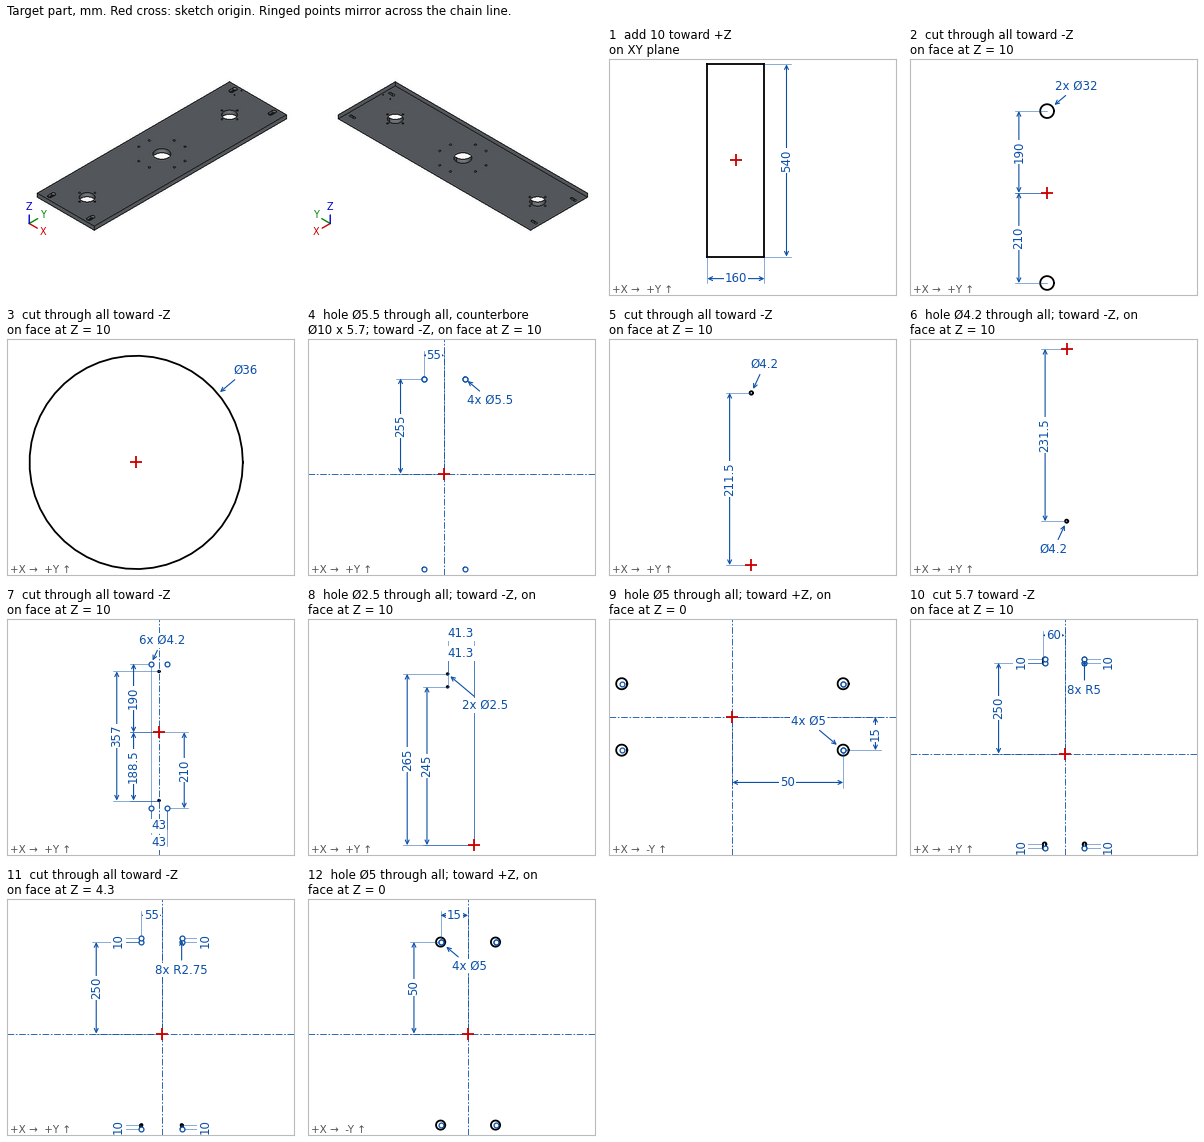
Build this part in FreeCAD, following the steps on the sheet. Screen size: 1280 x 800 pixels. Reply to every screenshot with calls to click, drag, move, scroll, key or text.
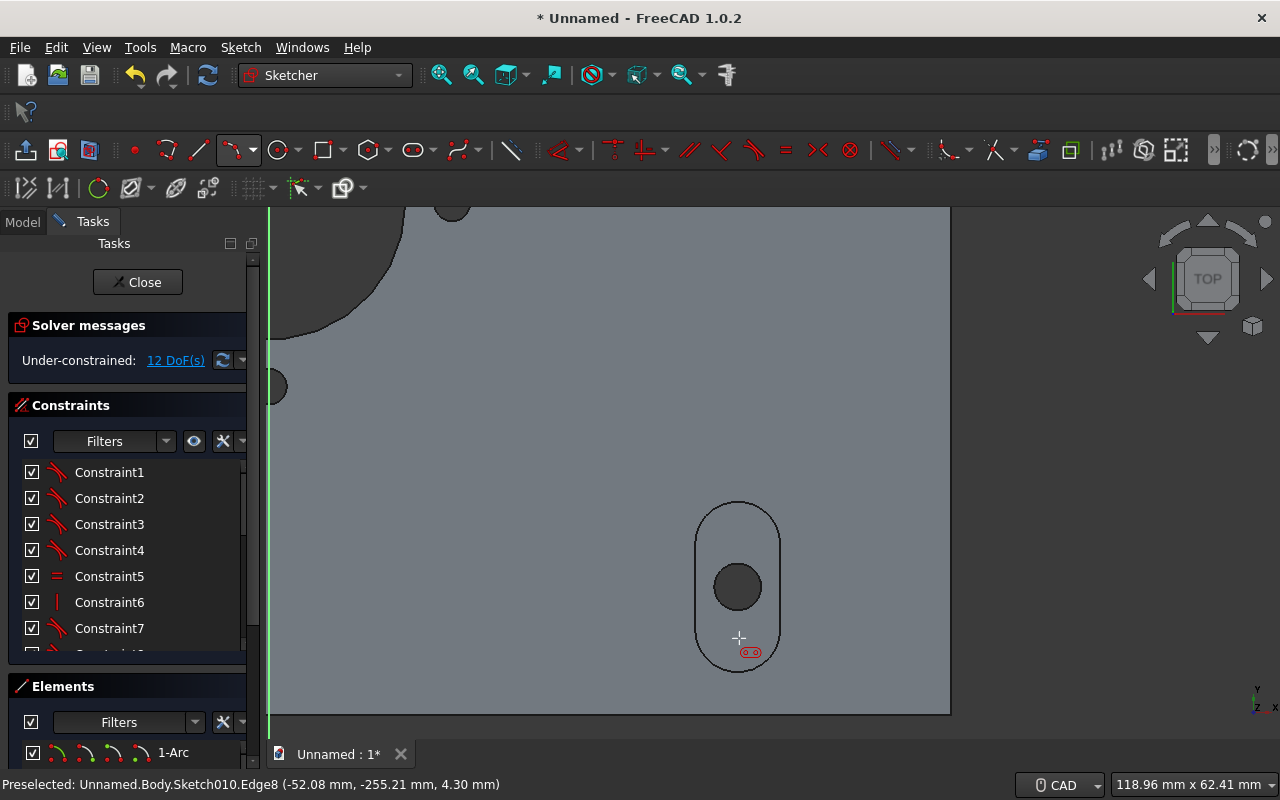
scroll(739, 638, down, 13)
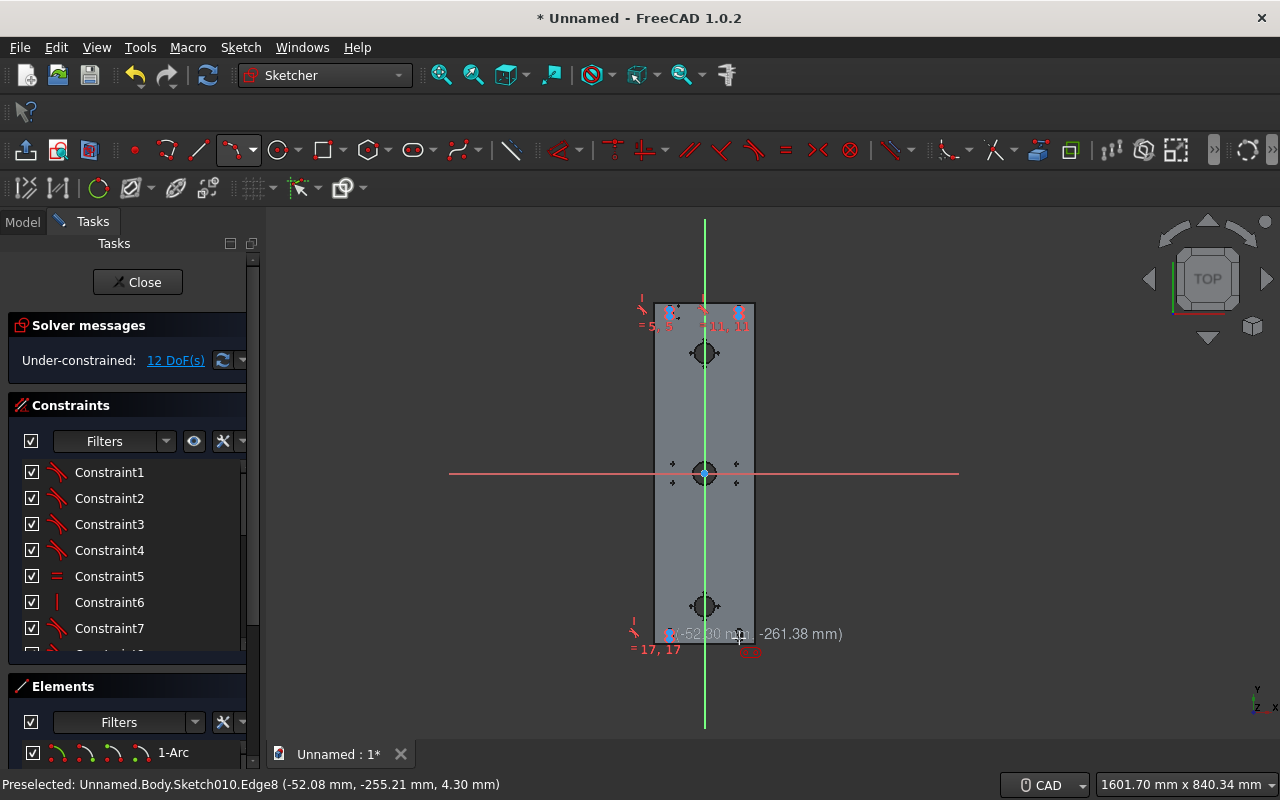
click(739, 638)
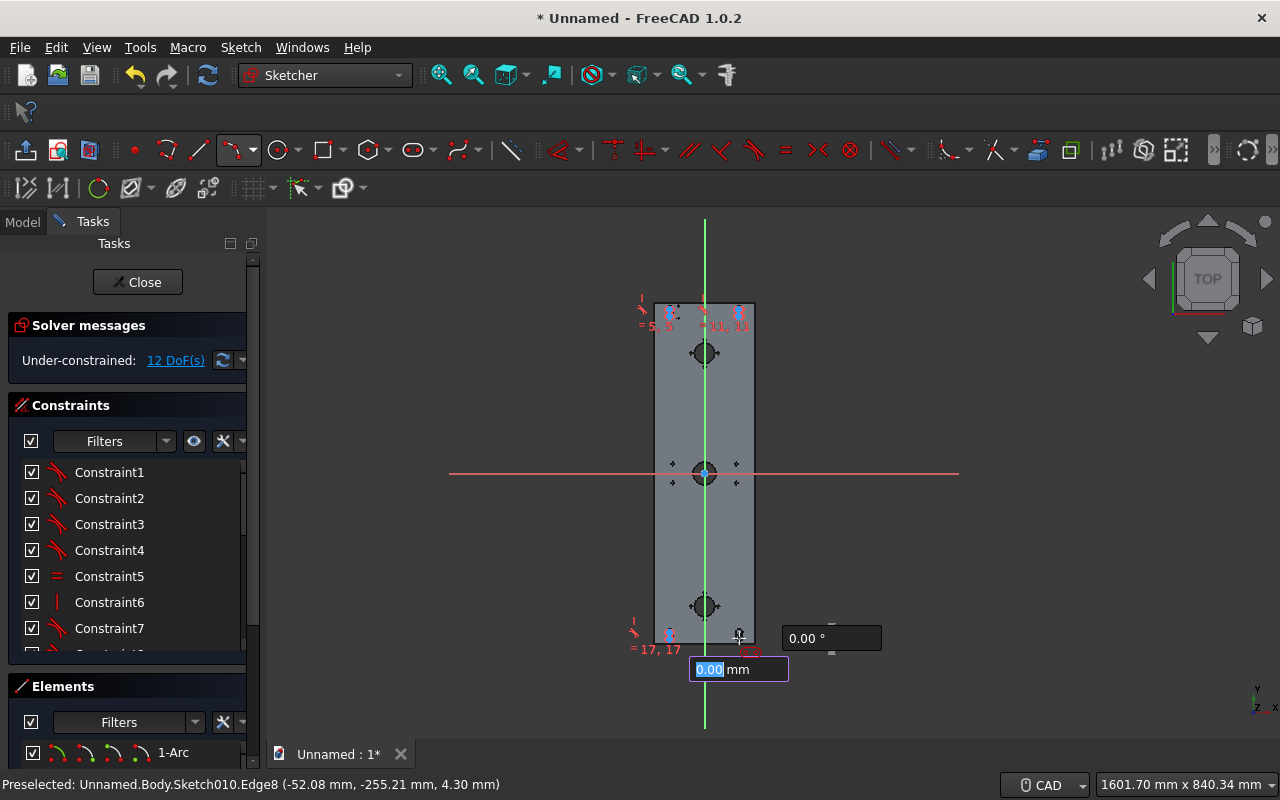
scroll(739, 632, up, 5)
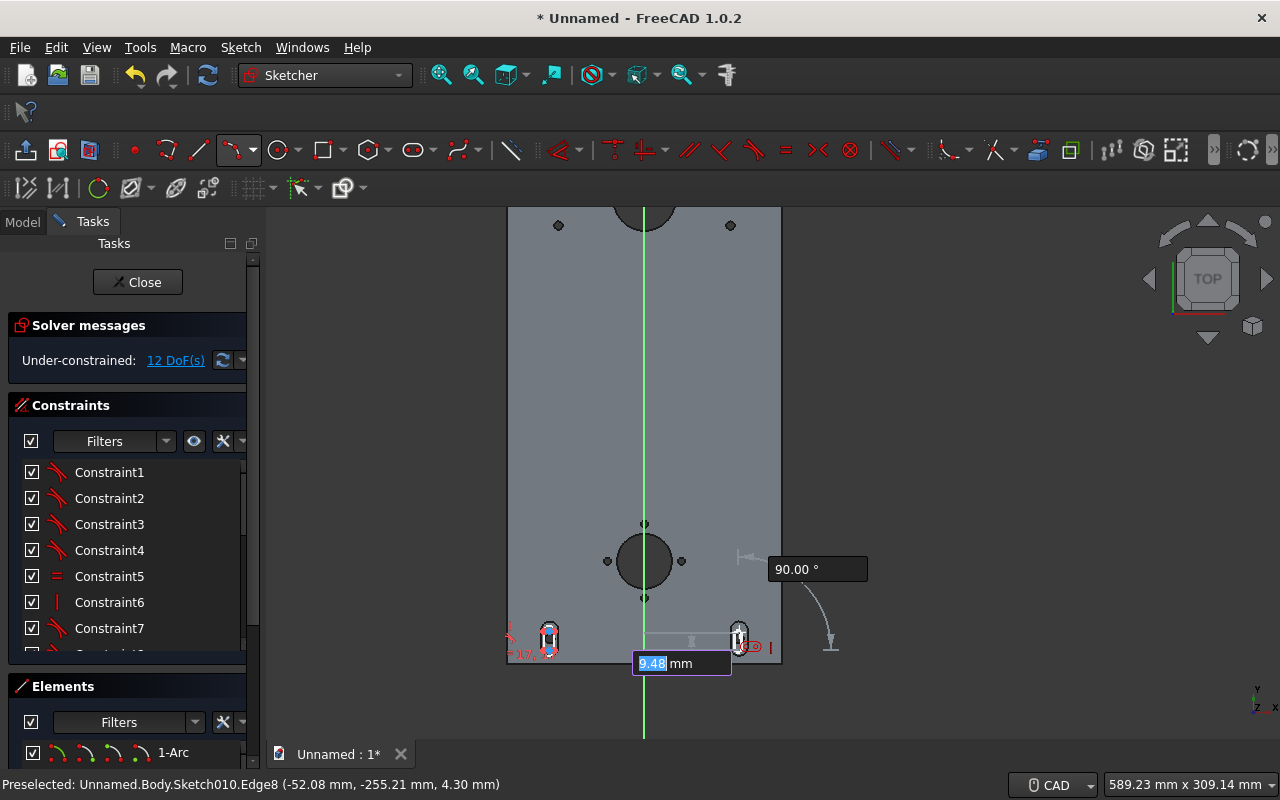
click(738, 630)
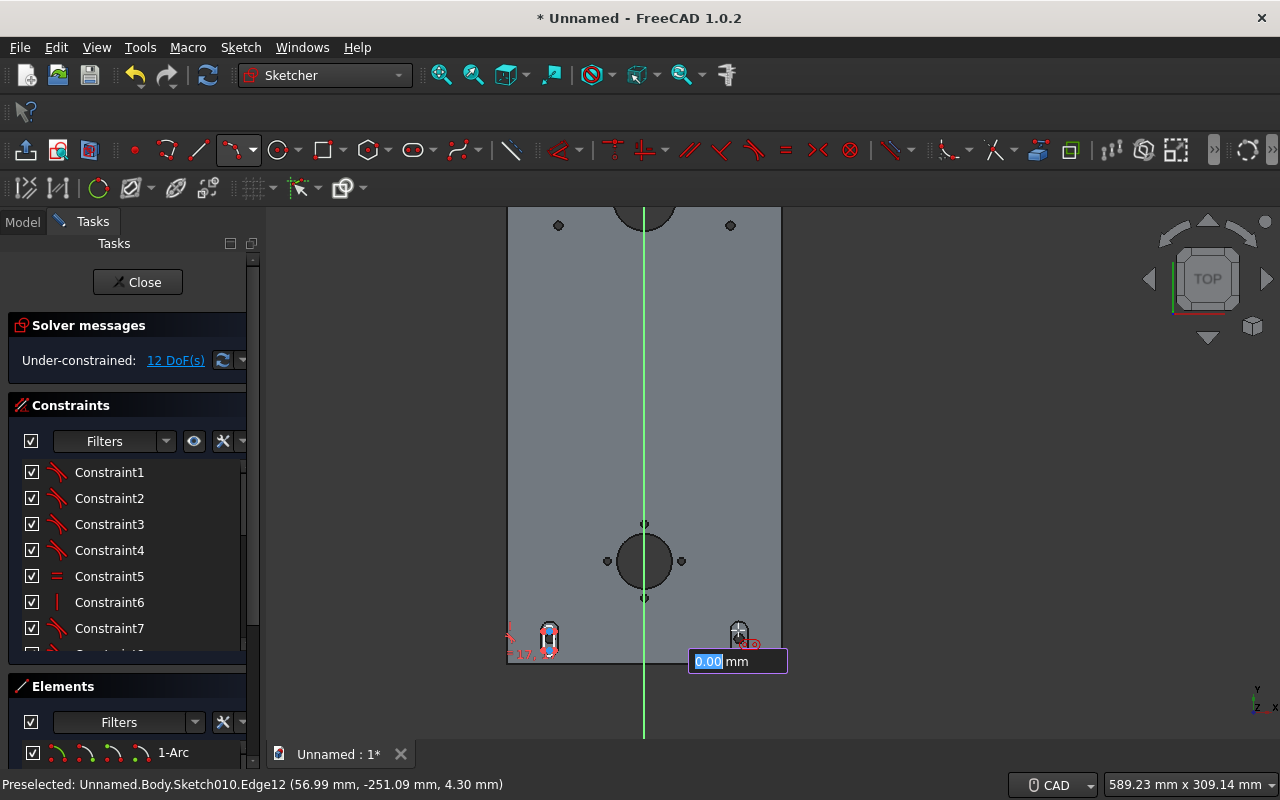
scroll(744, 639, up, 7)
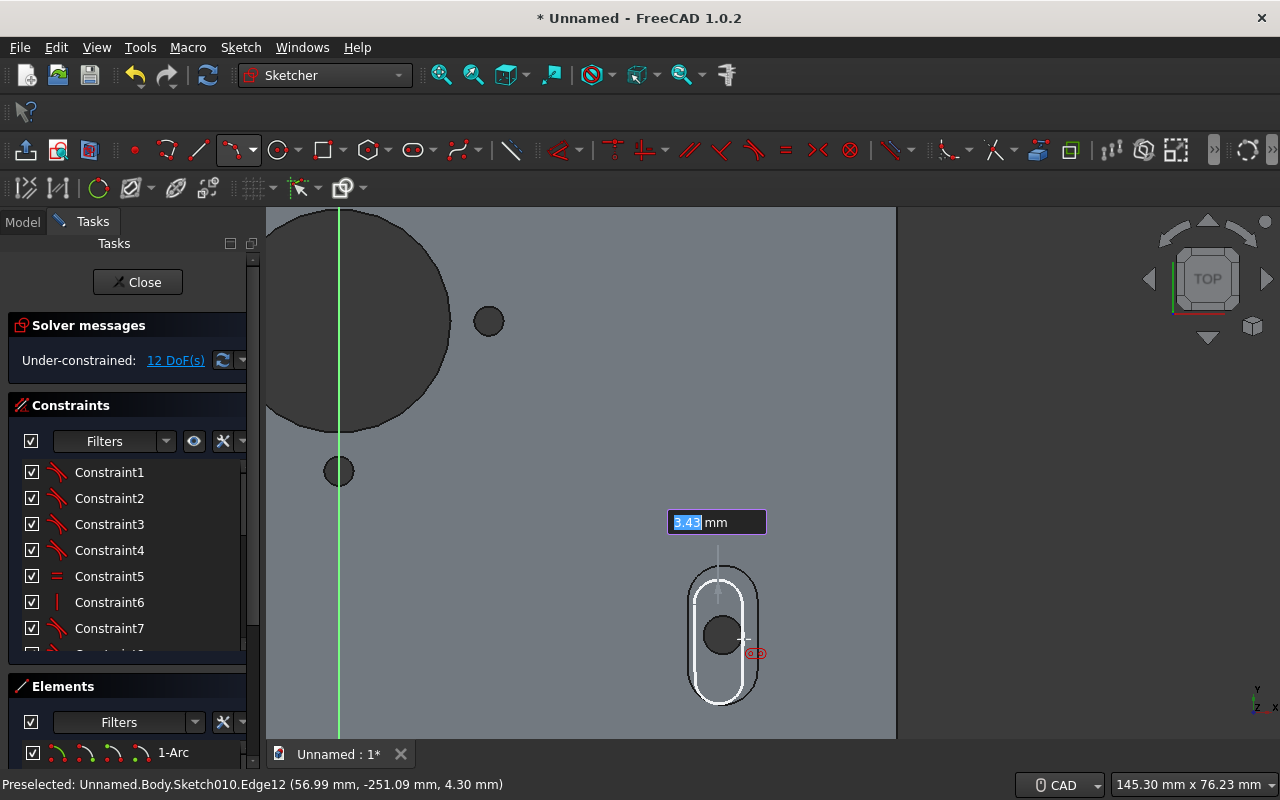
click(742, 635)
key(Escape)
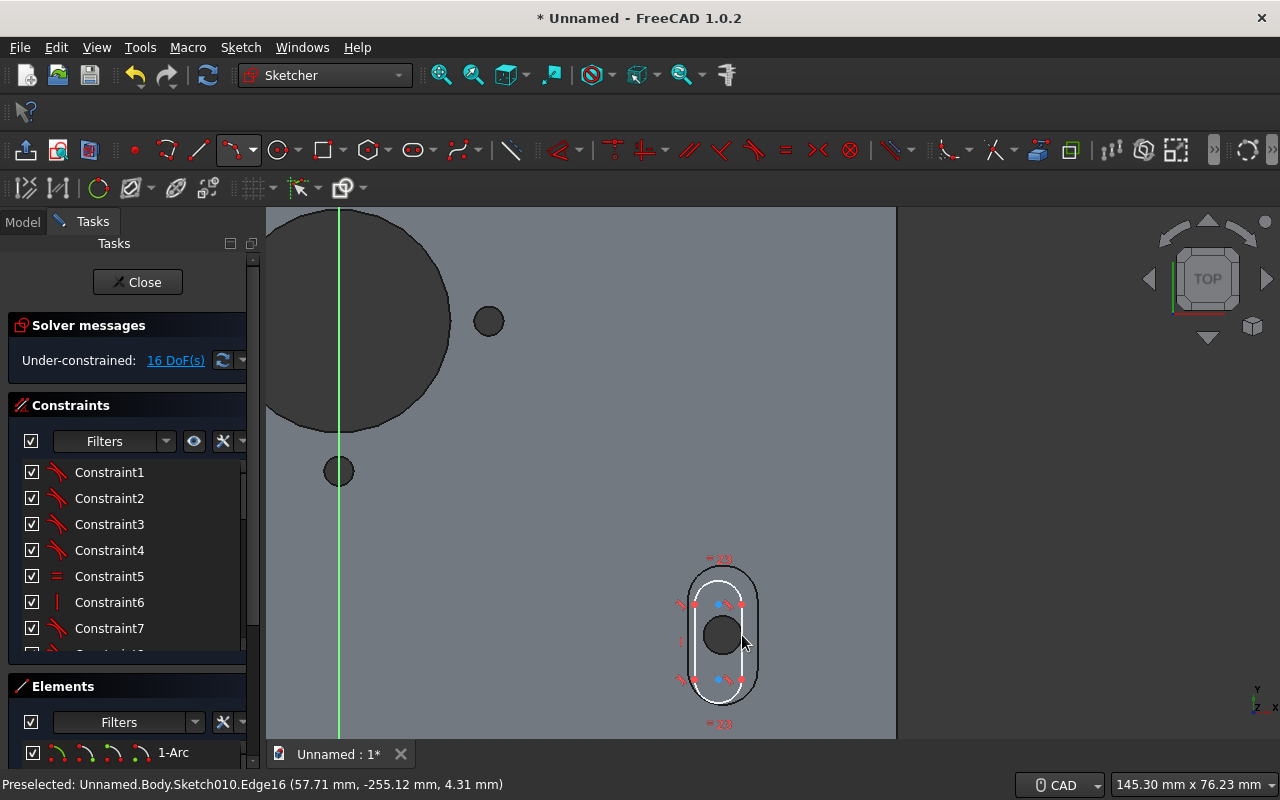
scroll(741, 634, down, 12)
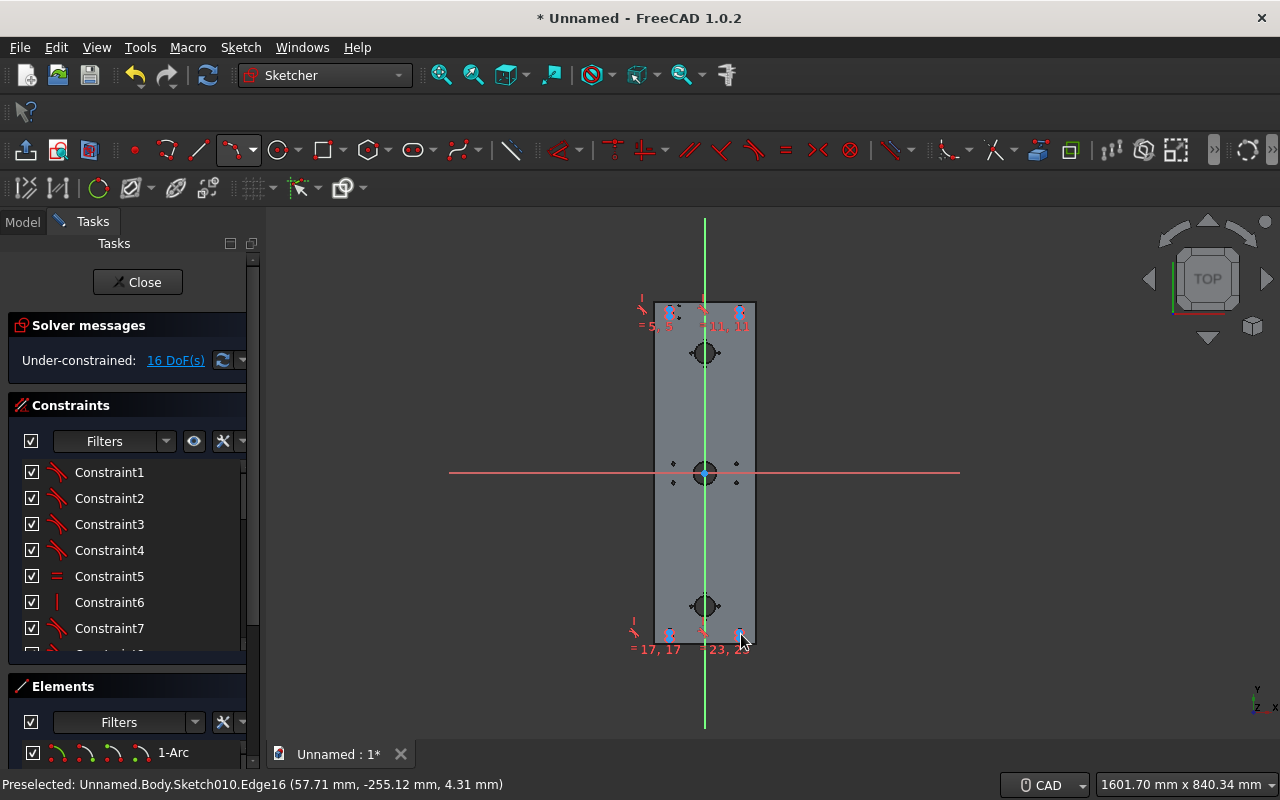
scroll(669, 318, up, 11)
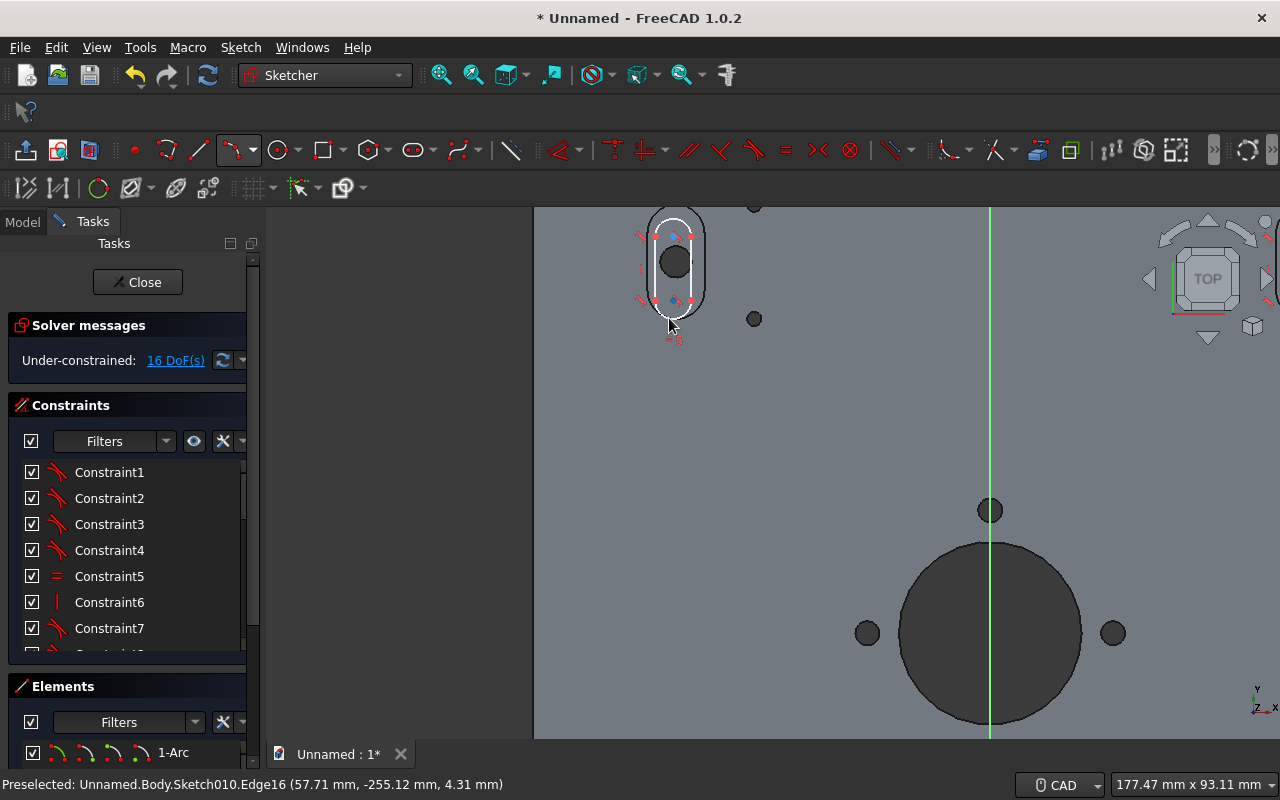
click(663, 315)